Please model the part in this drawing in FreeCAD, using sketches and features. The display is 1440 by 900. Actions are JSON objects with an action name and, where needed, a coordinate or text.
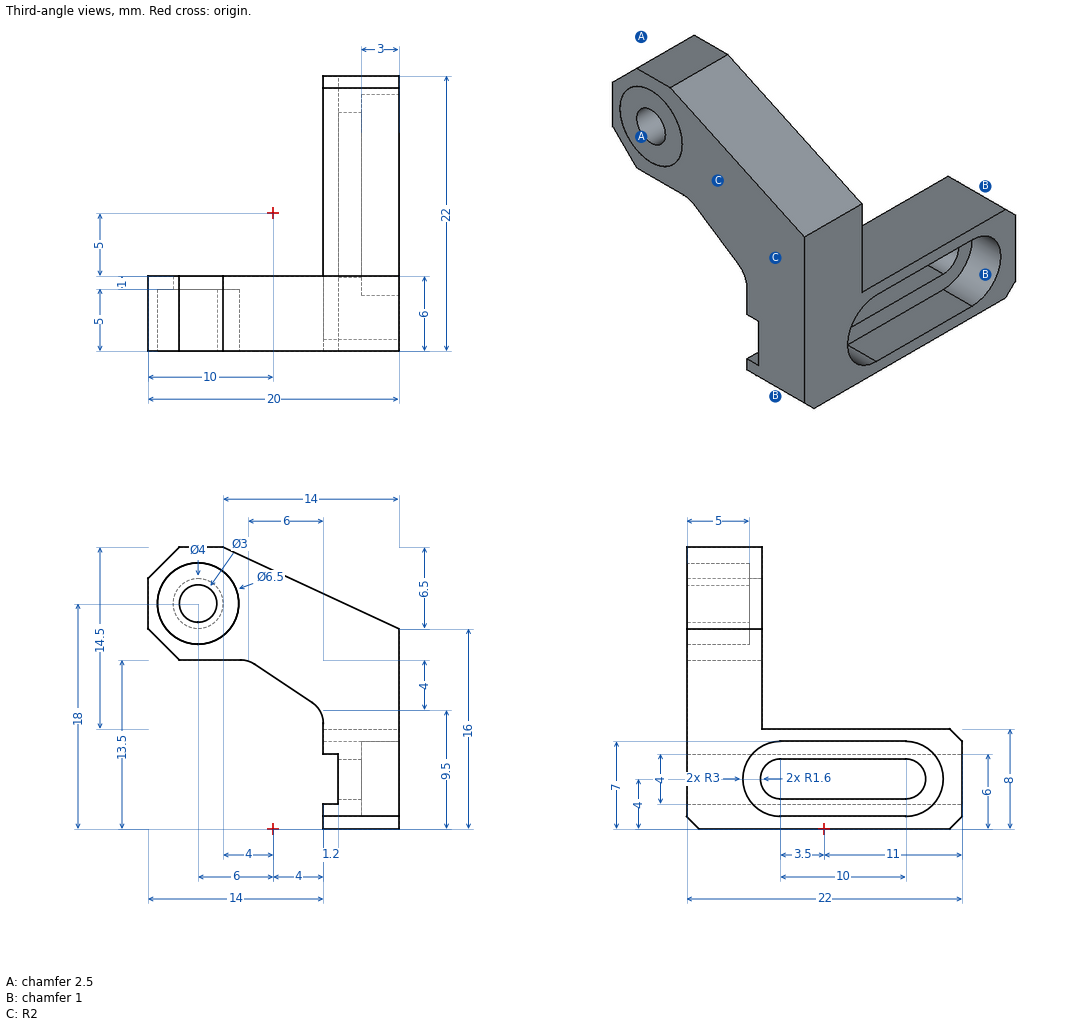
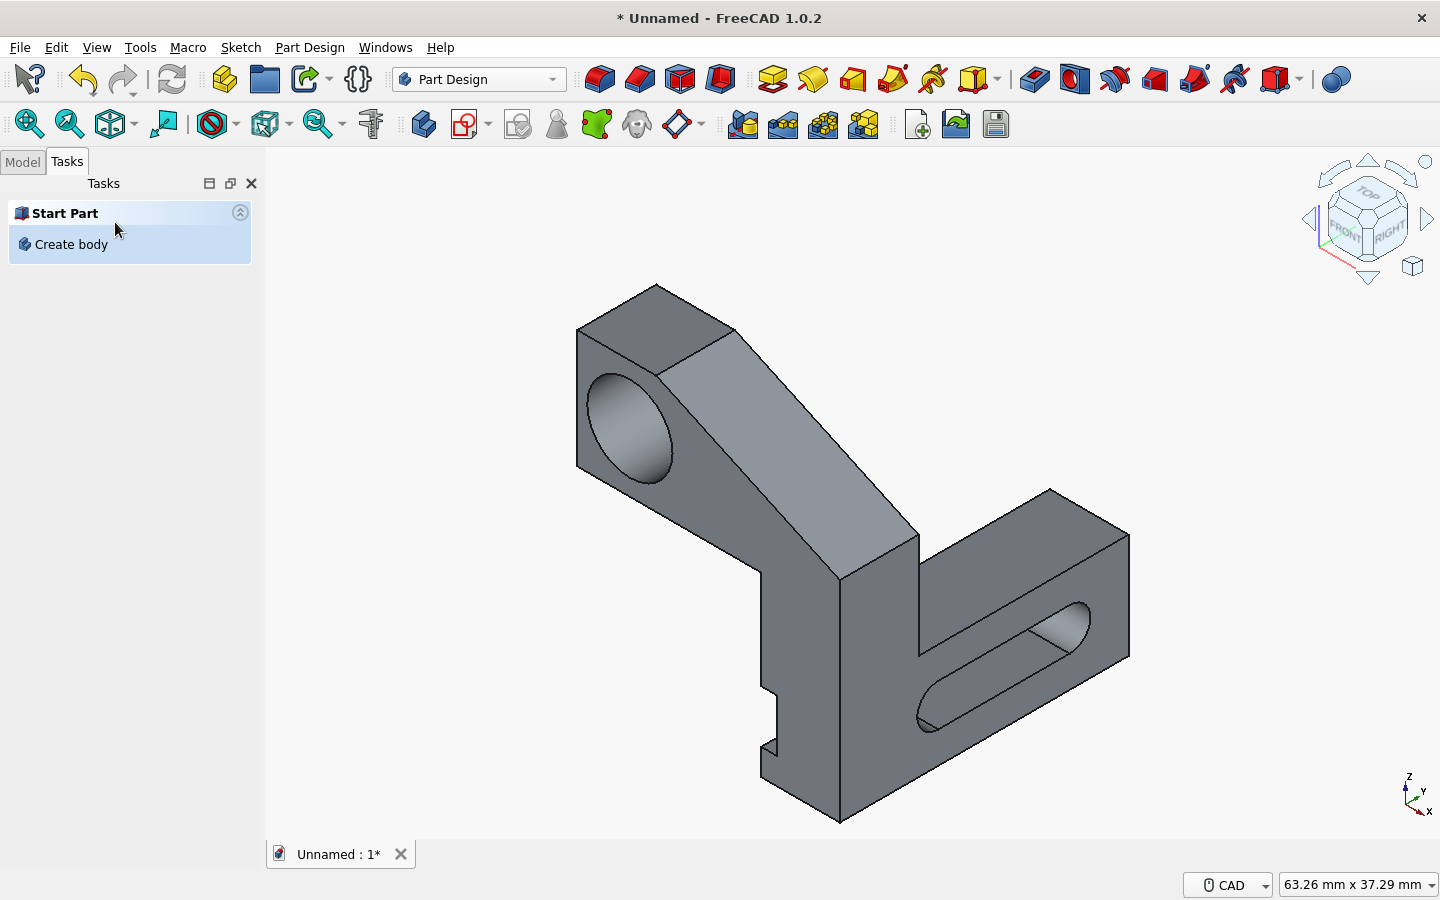
{"action": "left_click", "coordinate": [902, 699]}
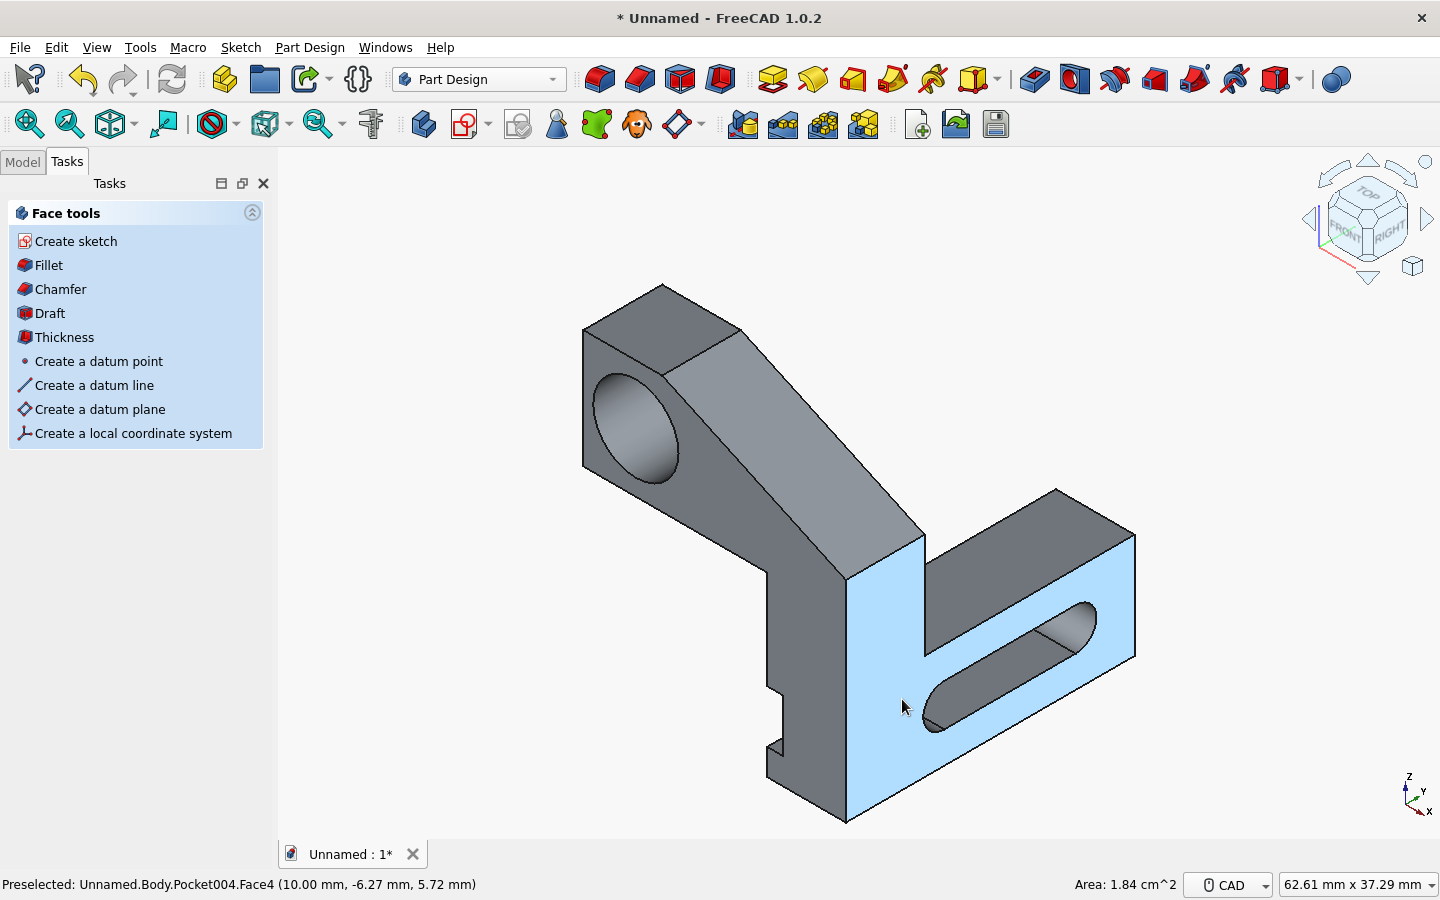
{"action": "left_click", "coordinate": [464, 124]}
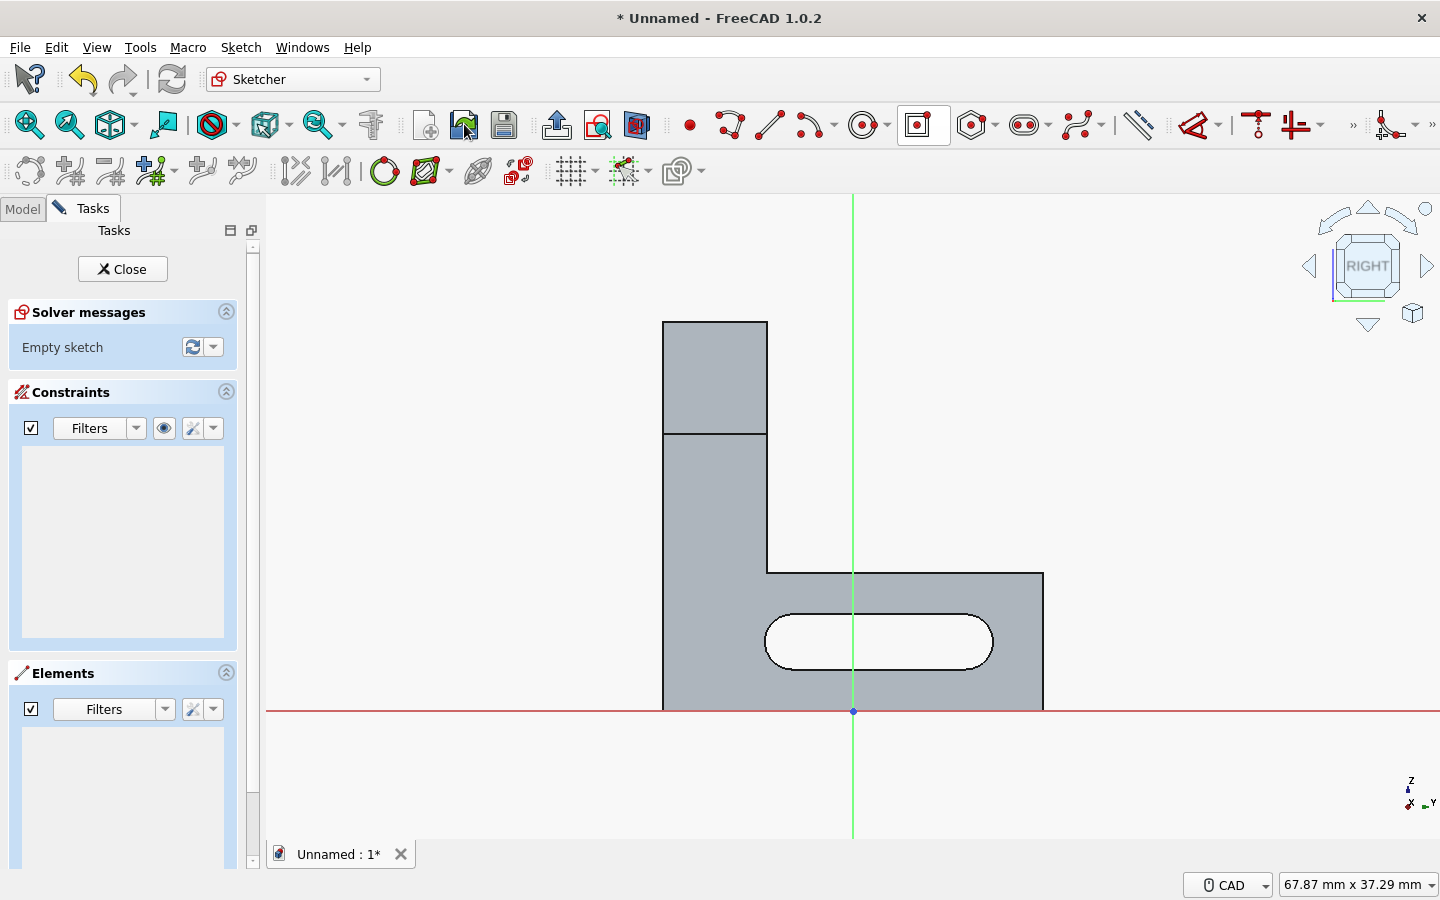
{"action": "scroll", "coordinate": [934, 729], "scroll_direction": "up", "scroll_amount": 5}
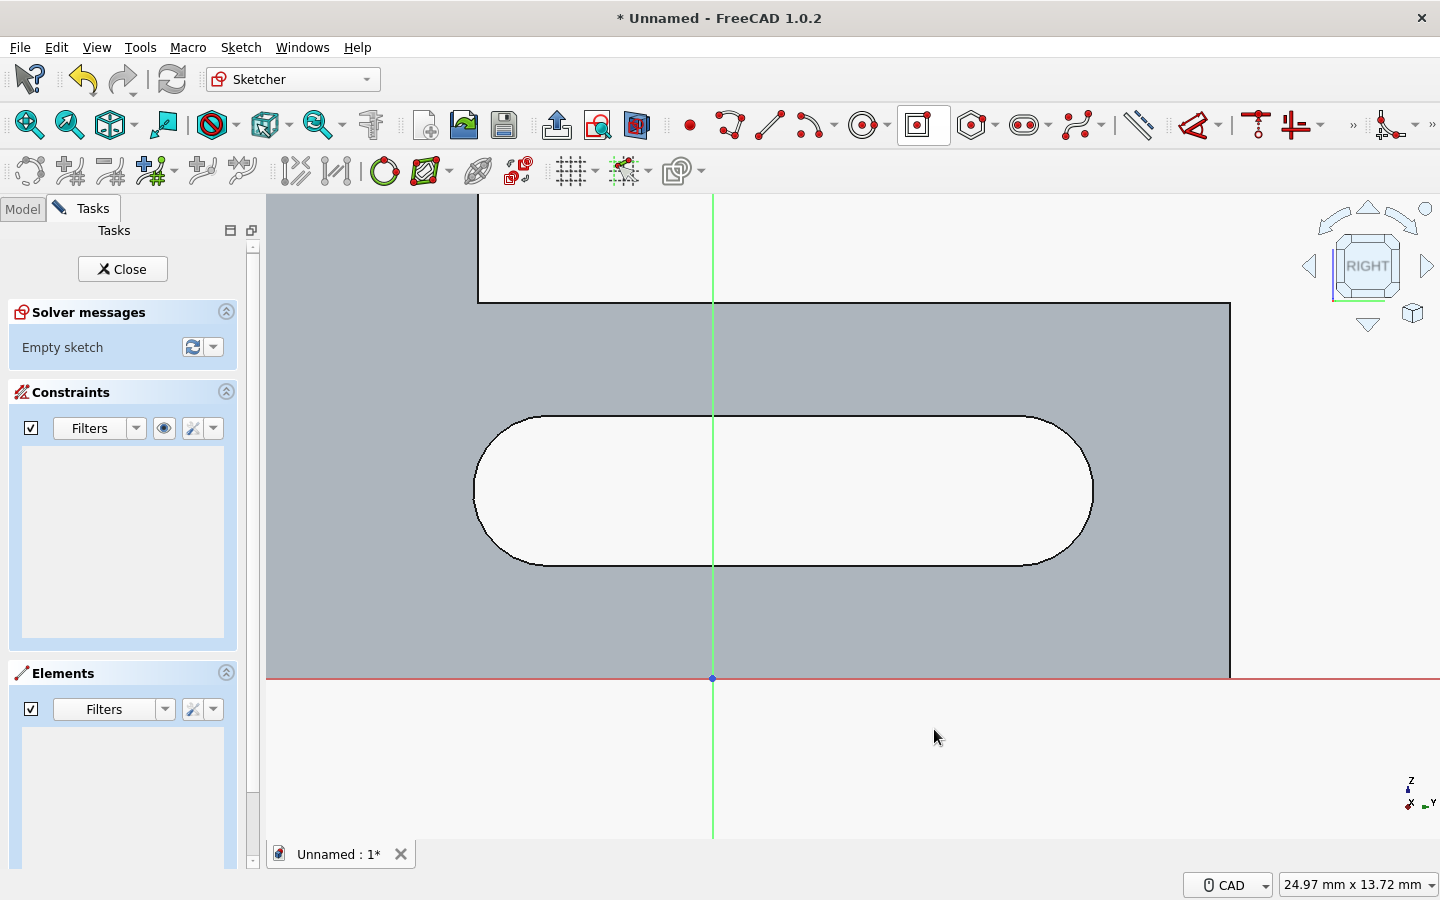
{"action": "left_click", "coordinate": [1024, 126]}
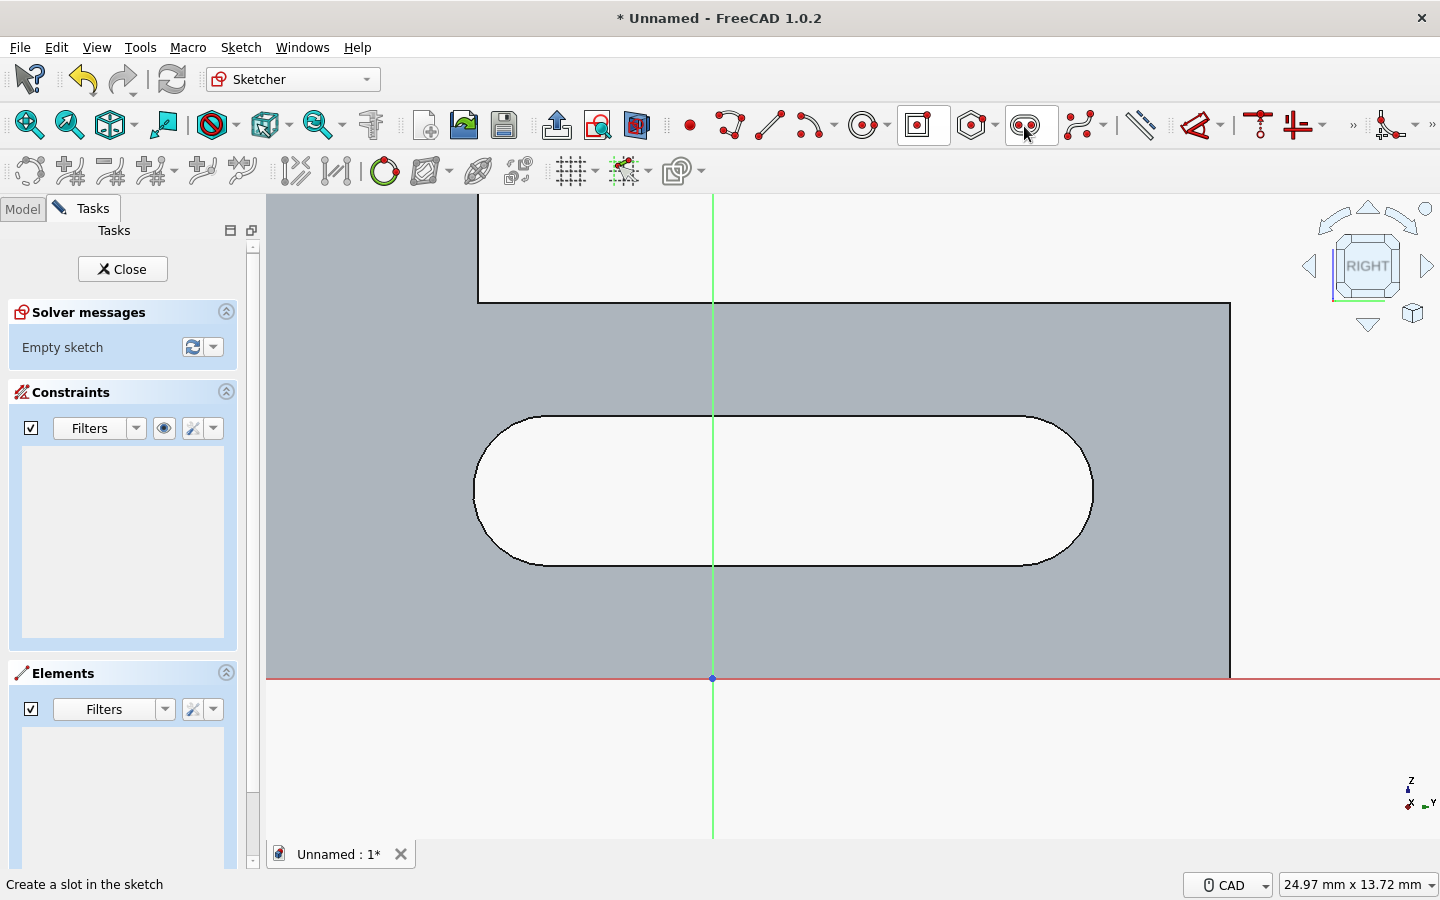
{"action": "left_click", "coordinate": [548, 491]}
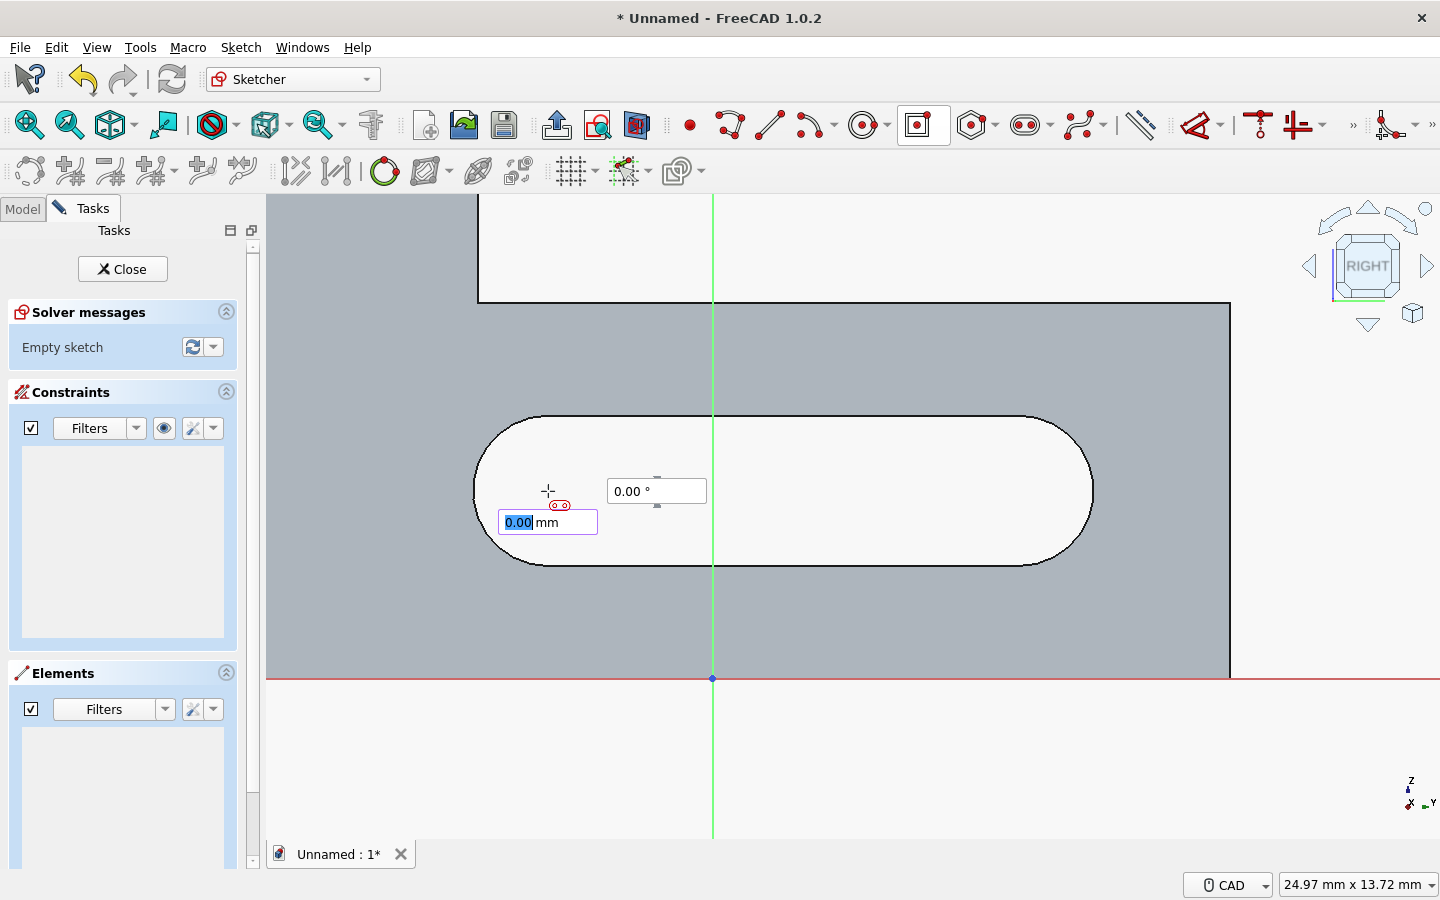
{"action": "left_click", "coordinate": [1018, 491]}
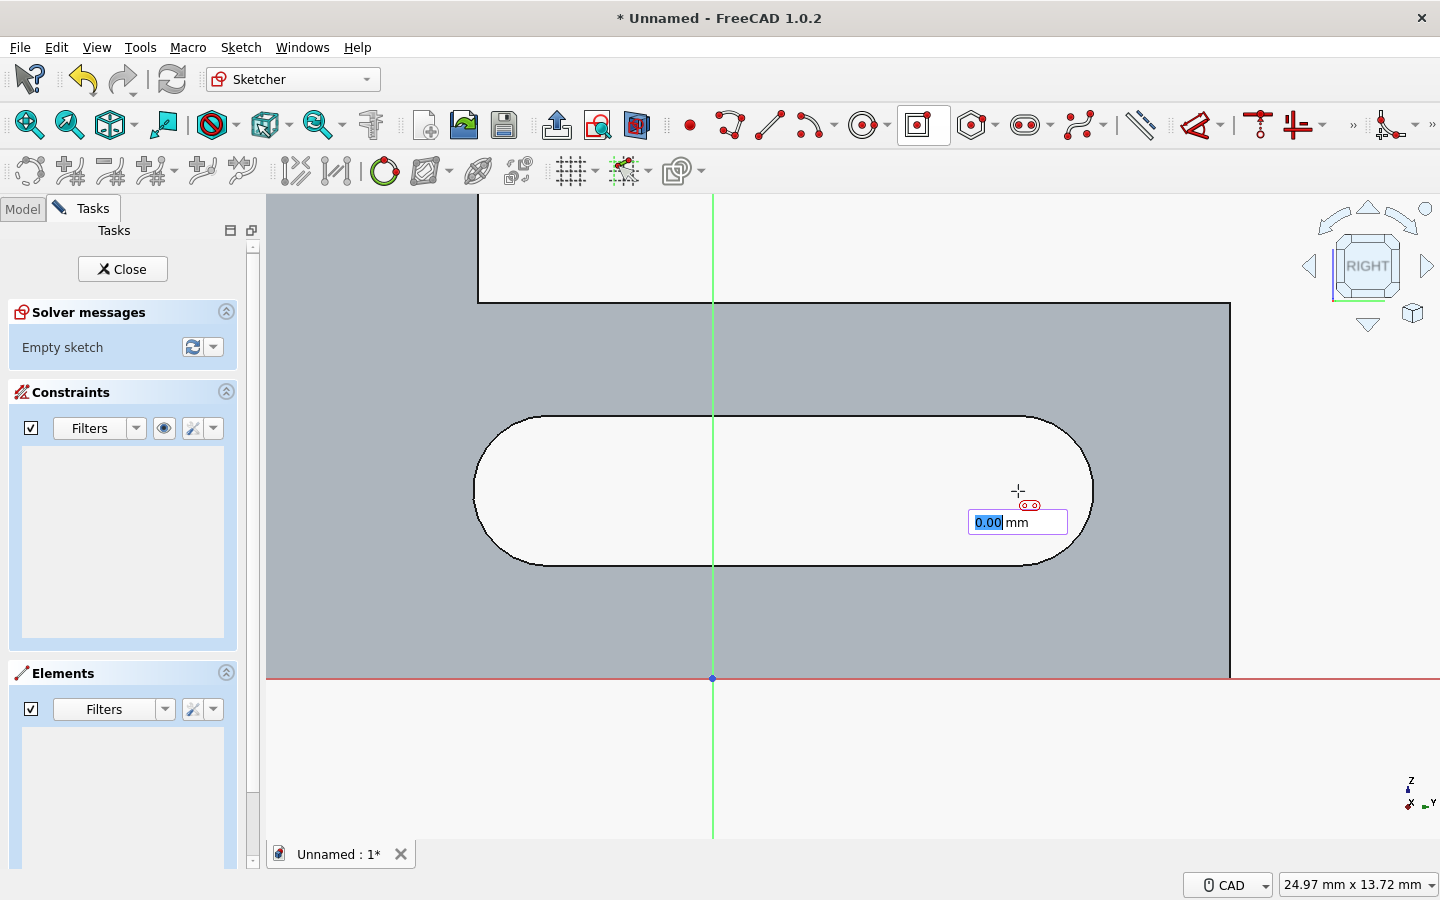
{"action": "left_click", "coordinate": [783, 350]}
{"action": "key", "text": "Escape"}